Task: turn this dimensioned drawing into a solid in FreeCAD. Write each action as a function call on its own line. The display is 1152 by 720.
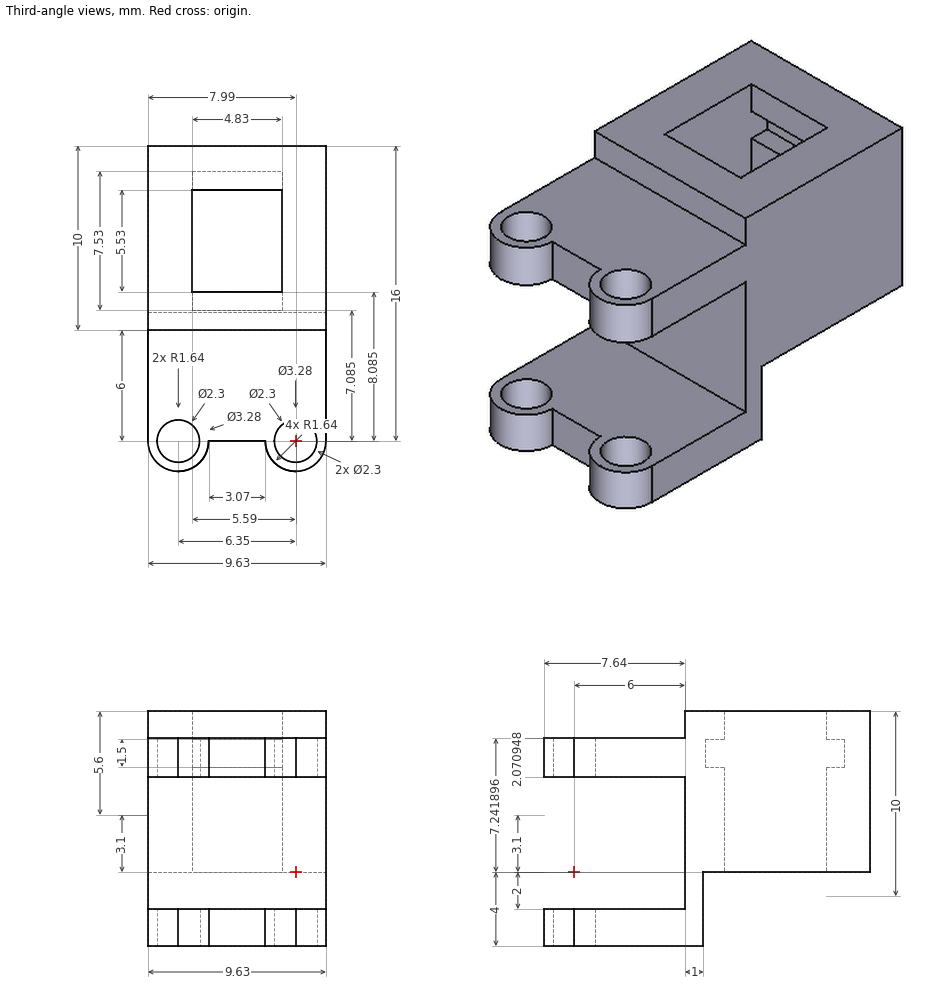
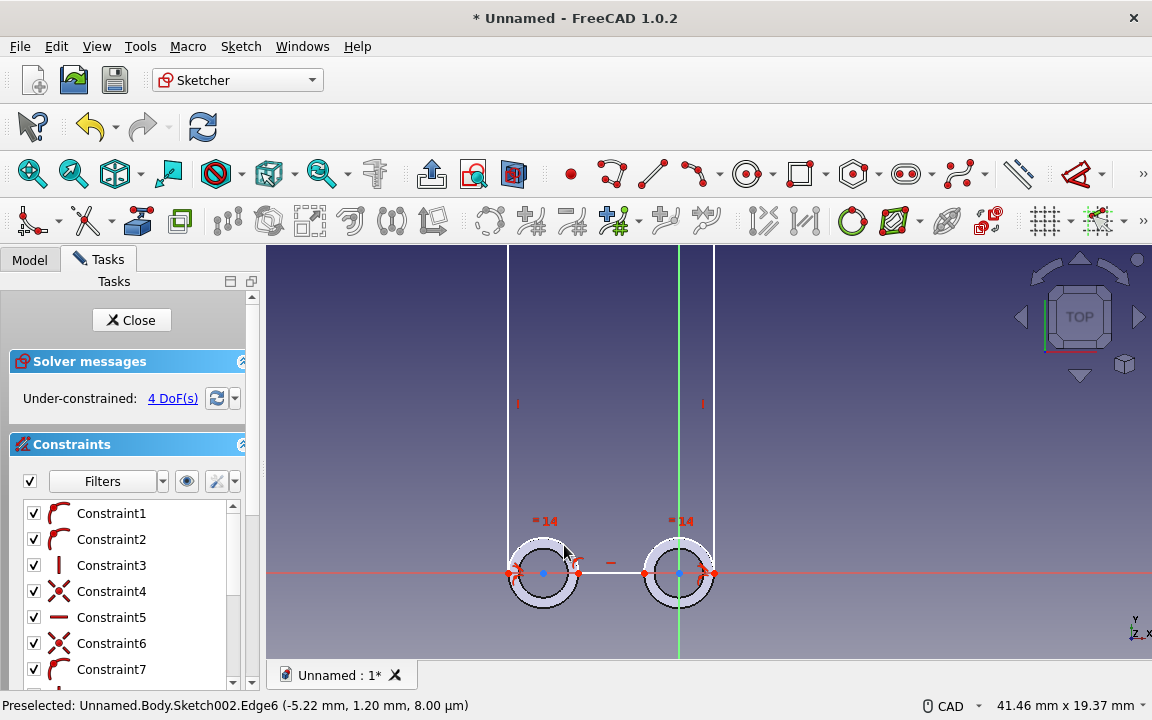
click(679, 573)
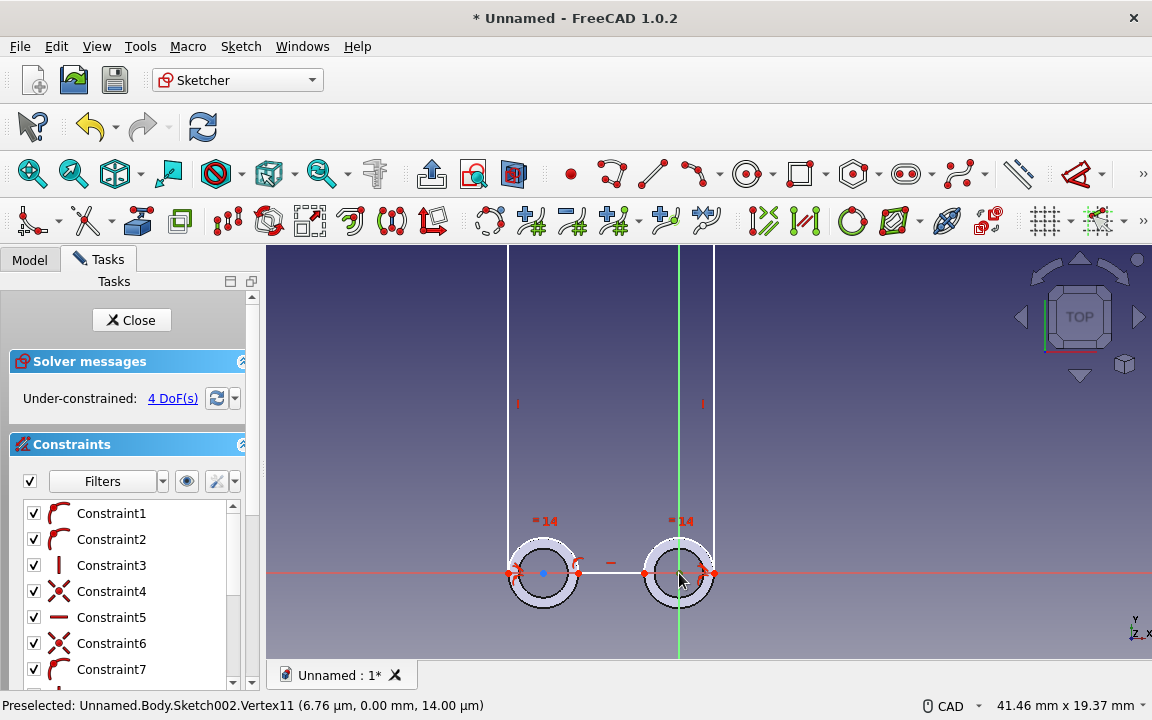
click(679, 605)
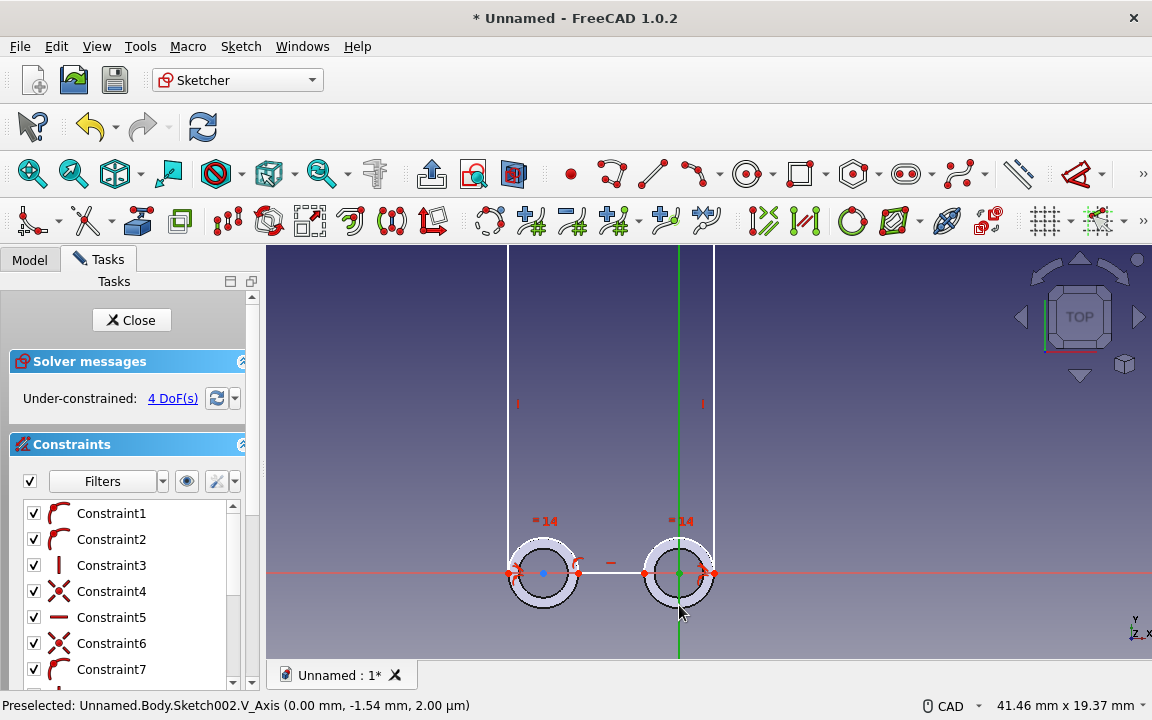
key(c)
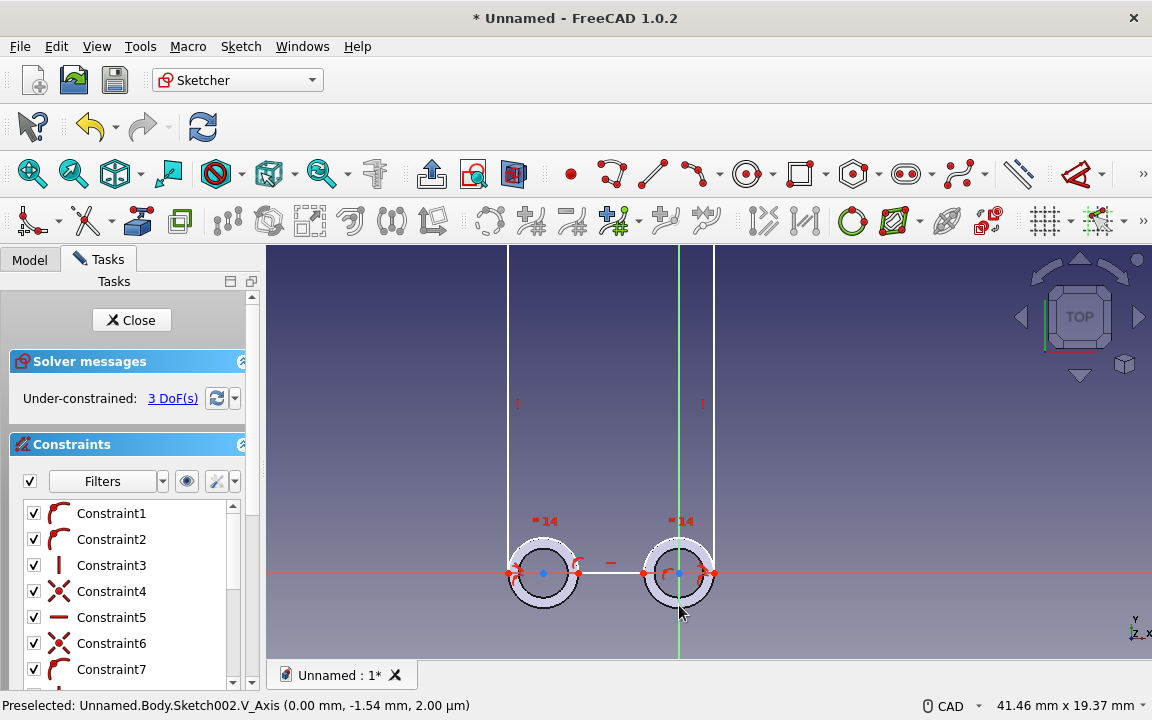
click(1076, 174)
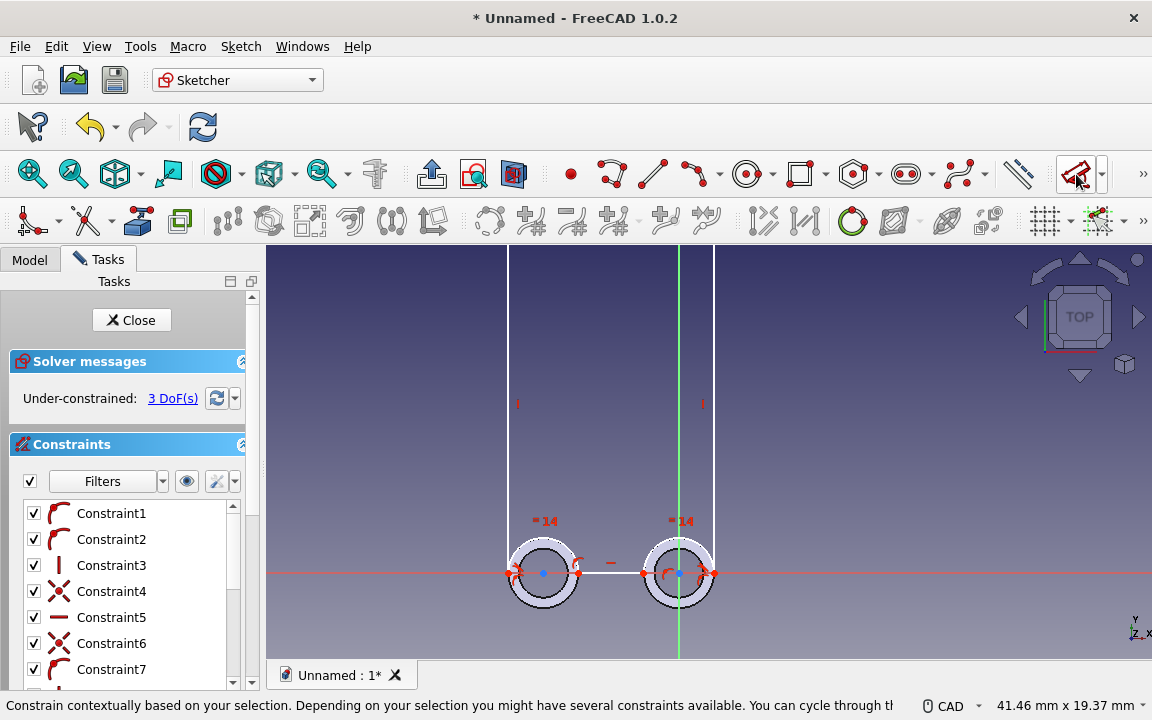
click(700, 545)
click(740, 545)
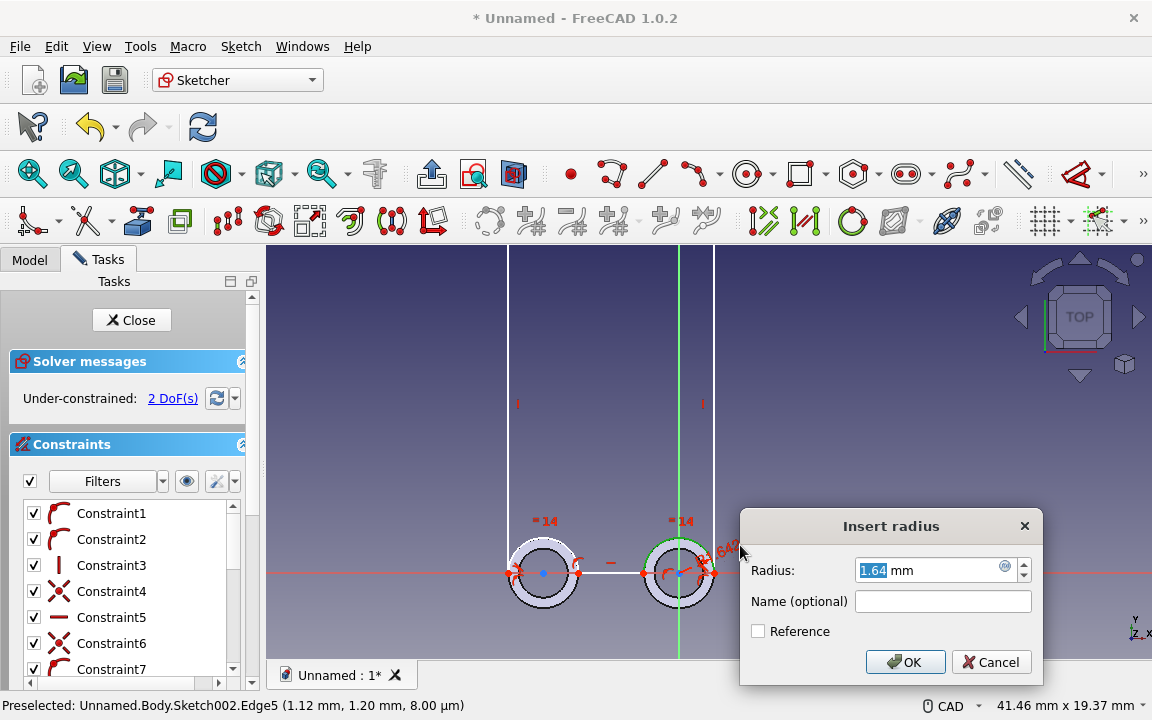
text(1.64)
key(Return)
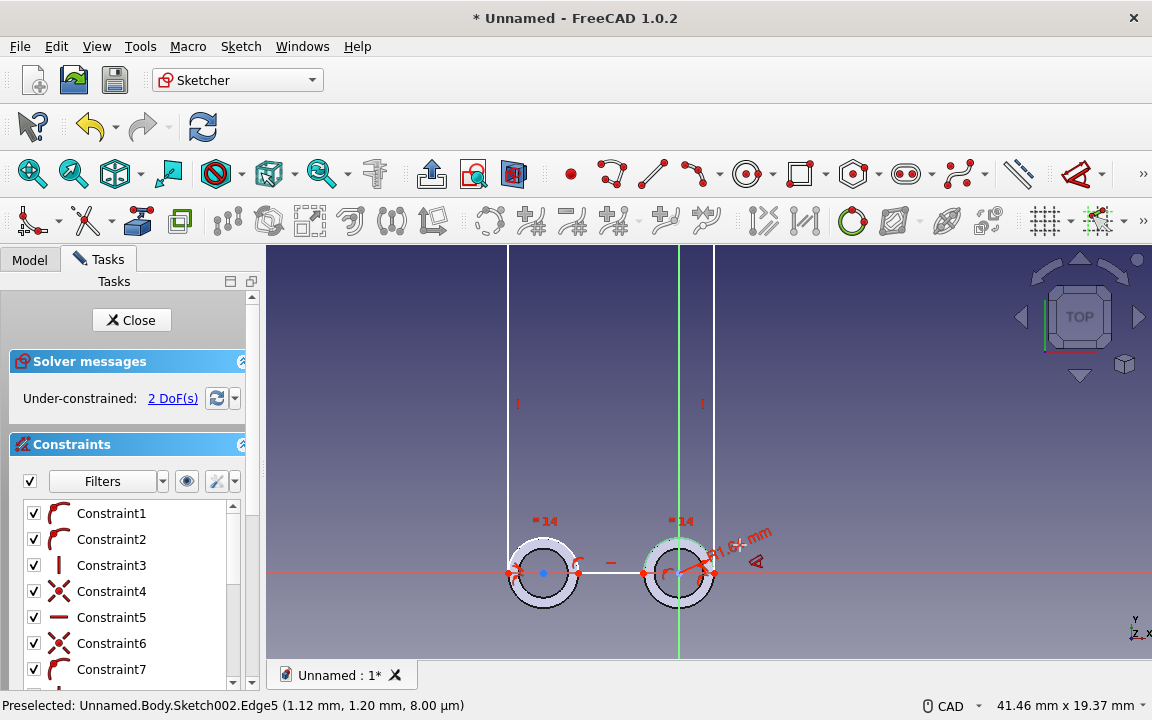
click(714, 471)
click(748, 423)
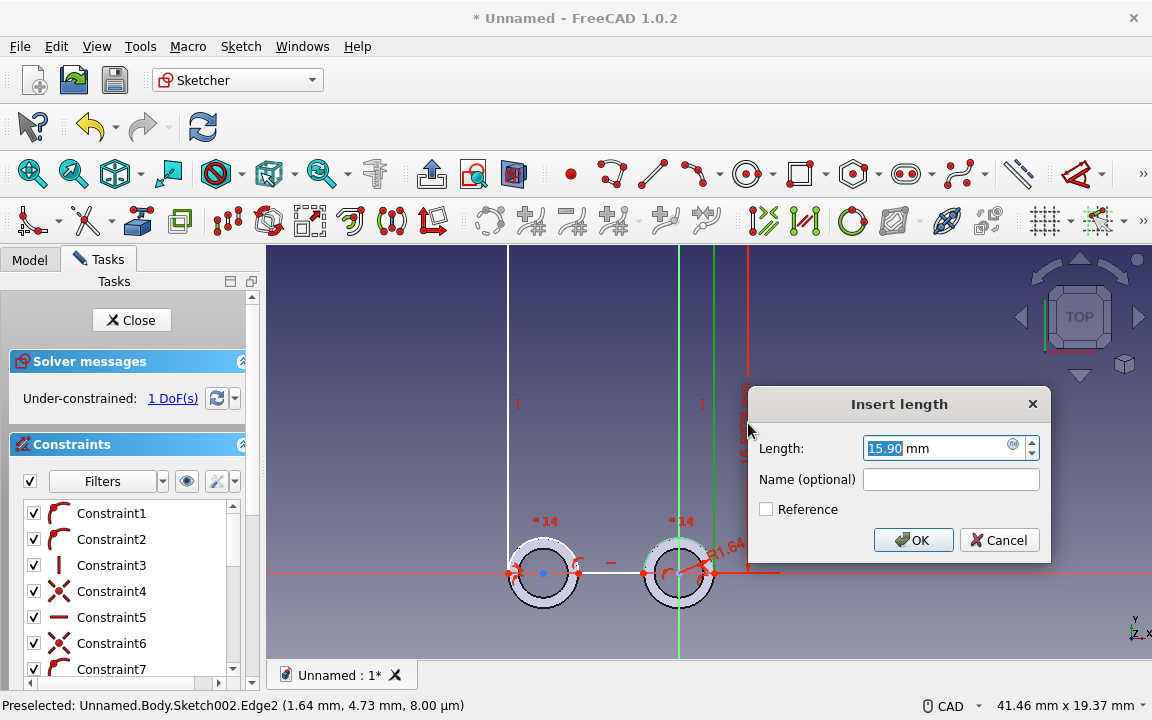
text(16)
key(Return)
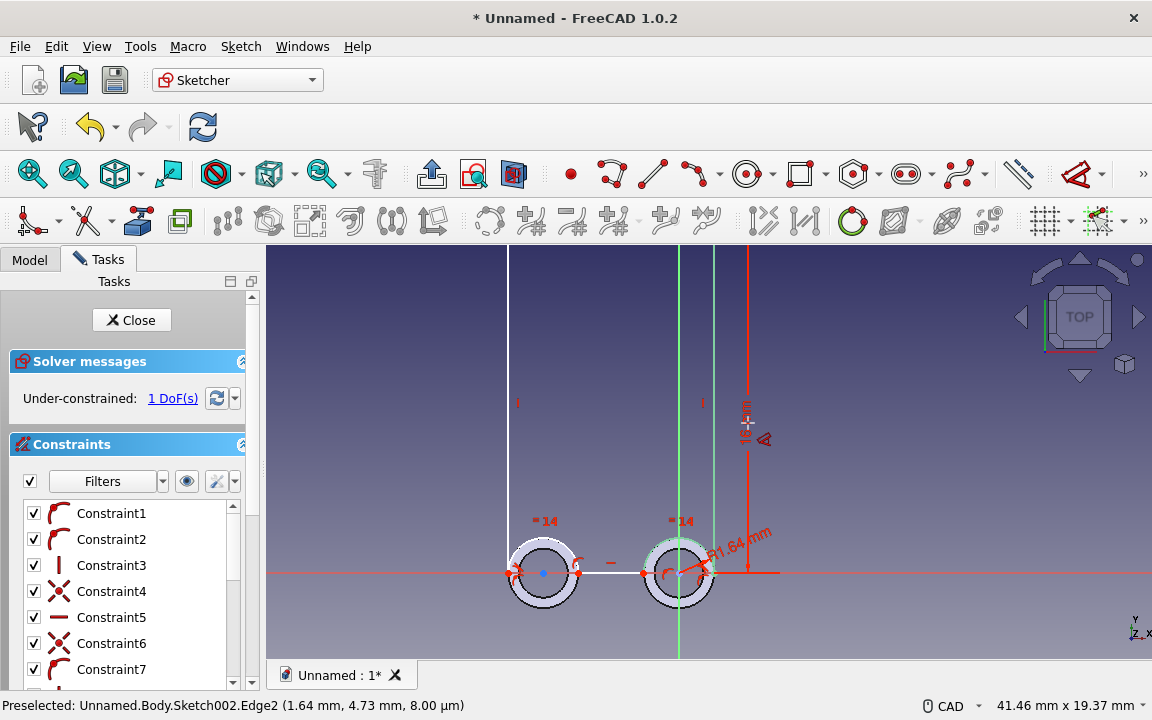
click(598, 573)
click(611, 607)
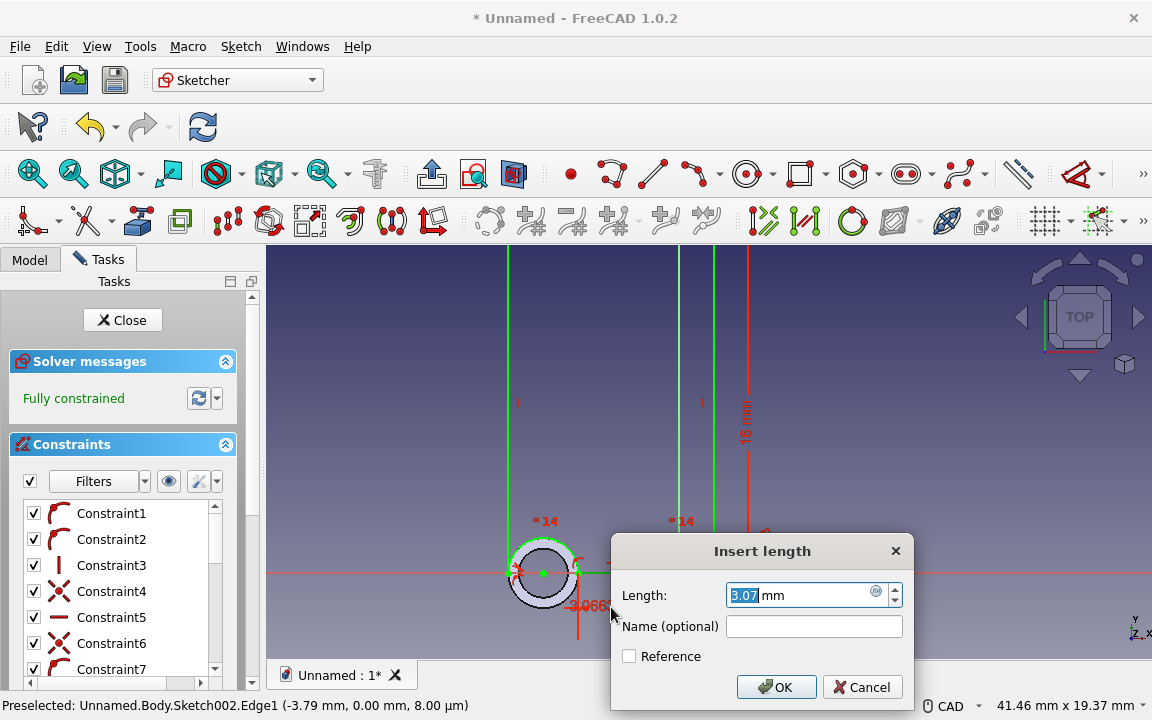
text(3.07)
key(Return)
key(Escape)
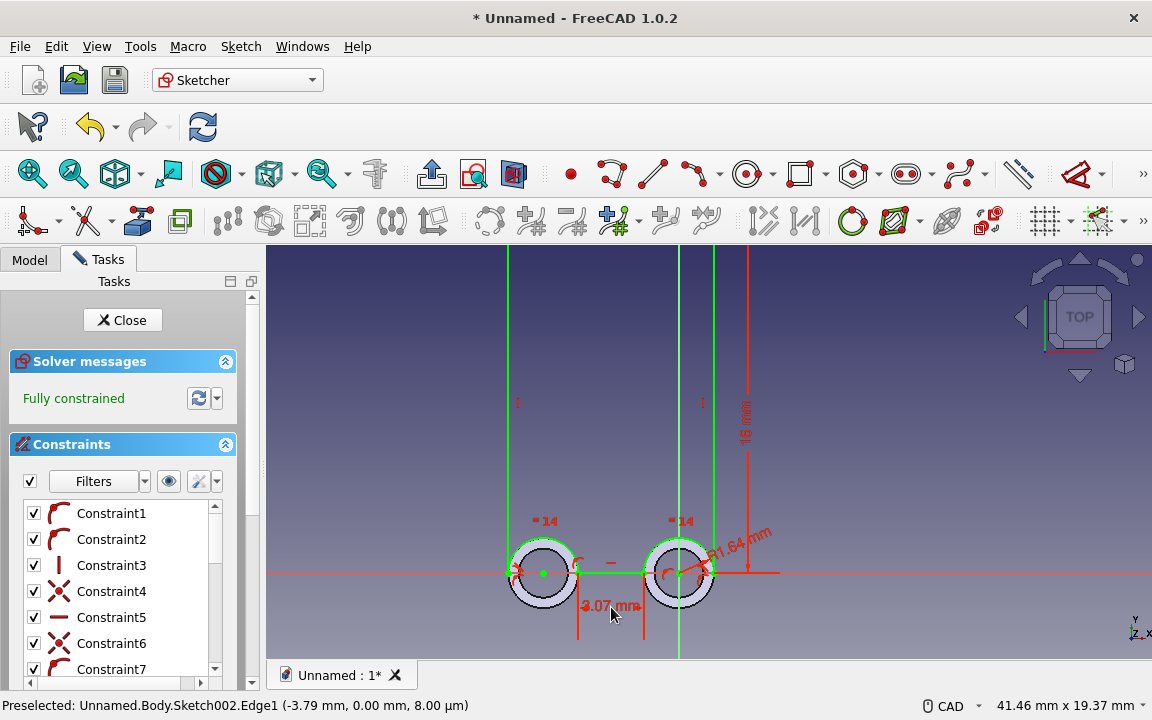
click(123, 320)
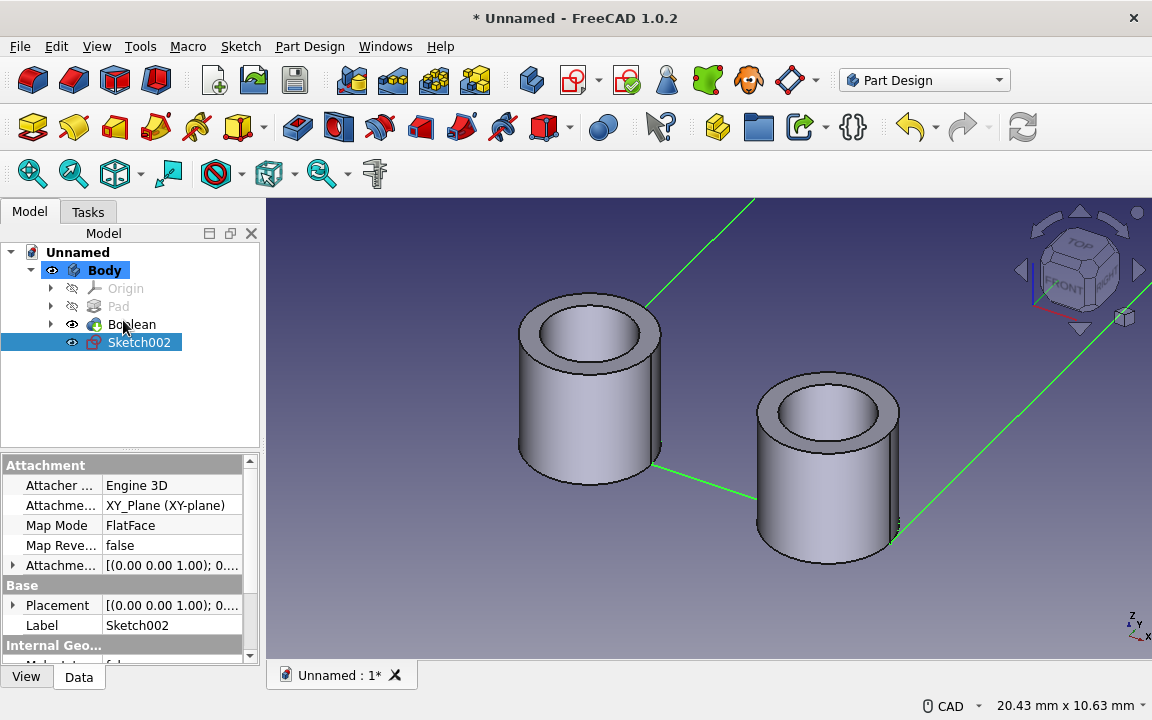
click(33, 128)